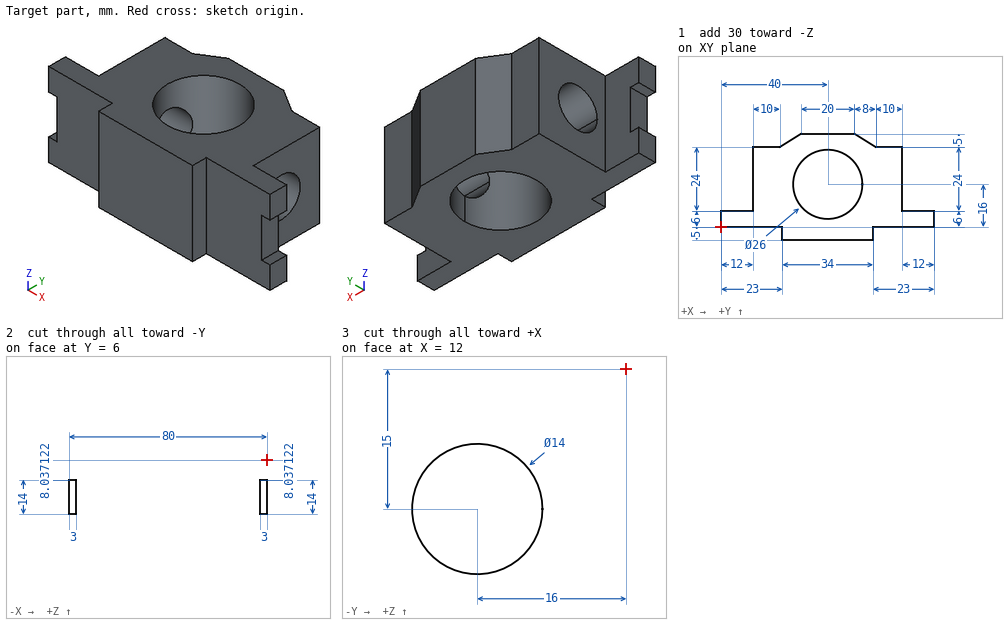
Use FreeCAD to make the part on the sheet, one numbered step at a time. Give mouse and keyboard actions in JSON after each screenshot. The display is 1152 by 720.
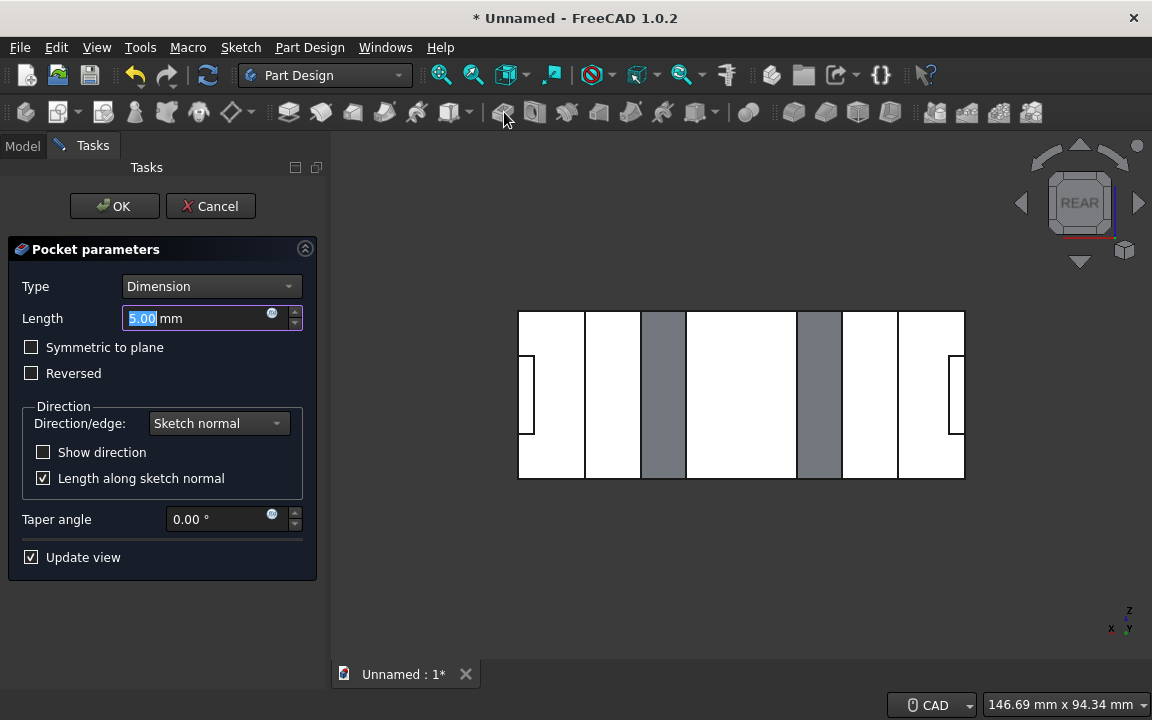
{"action": "left_click", "coordinate": [212, 286]}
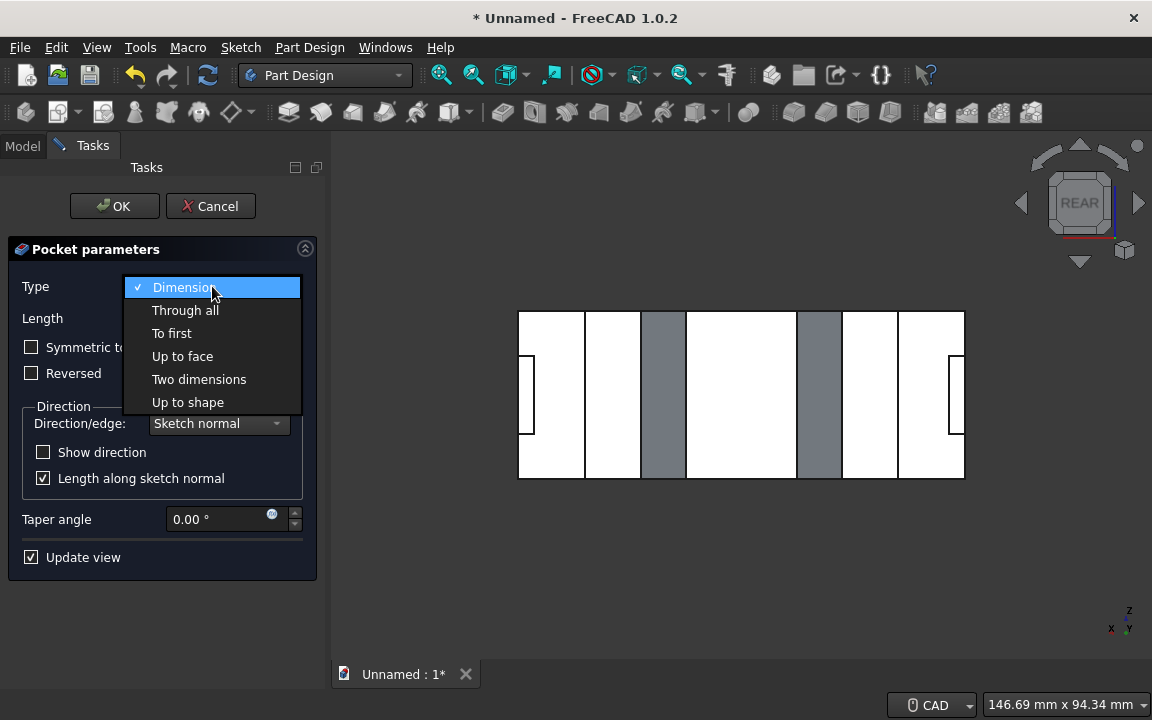
{"action": "left_click", "coordinate": [212, 310]}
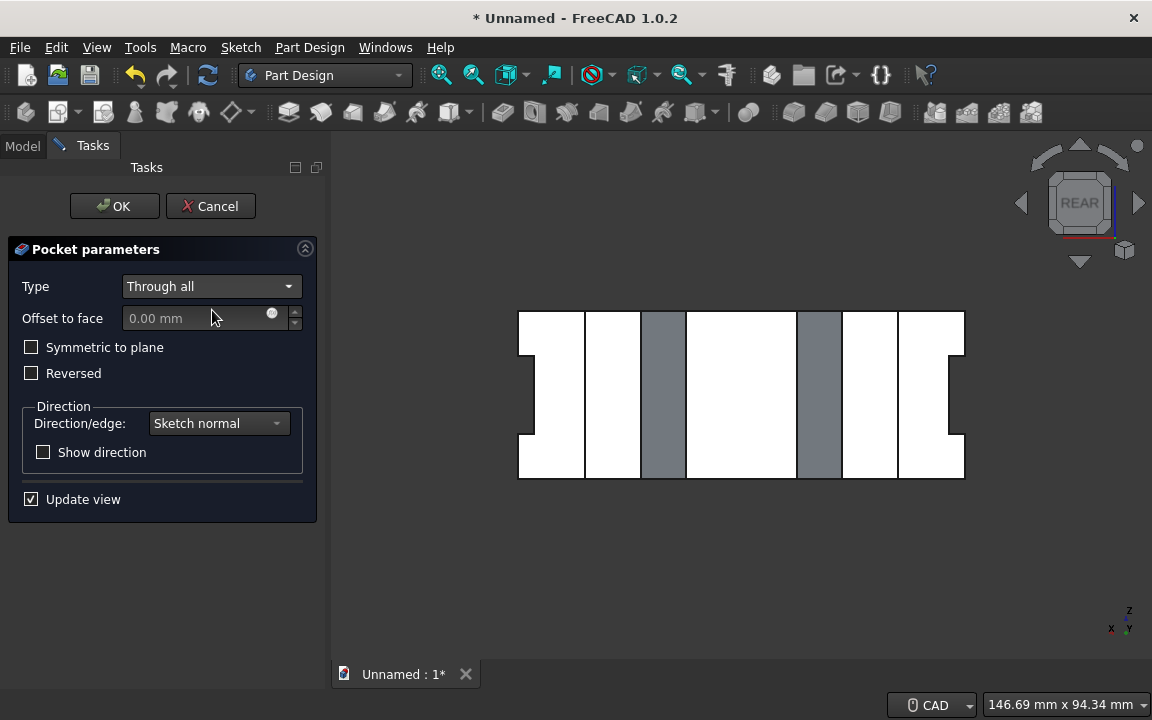
{"action": "left_click", "coordinate": [115, 206]}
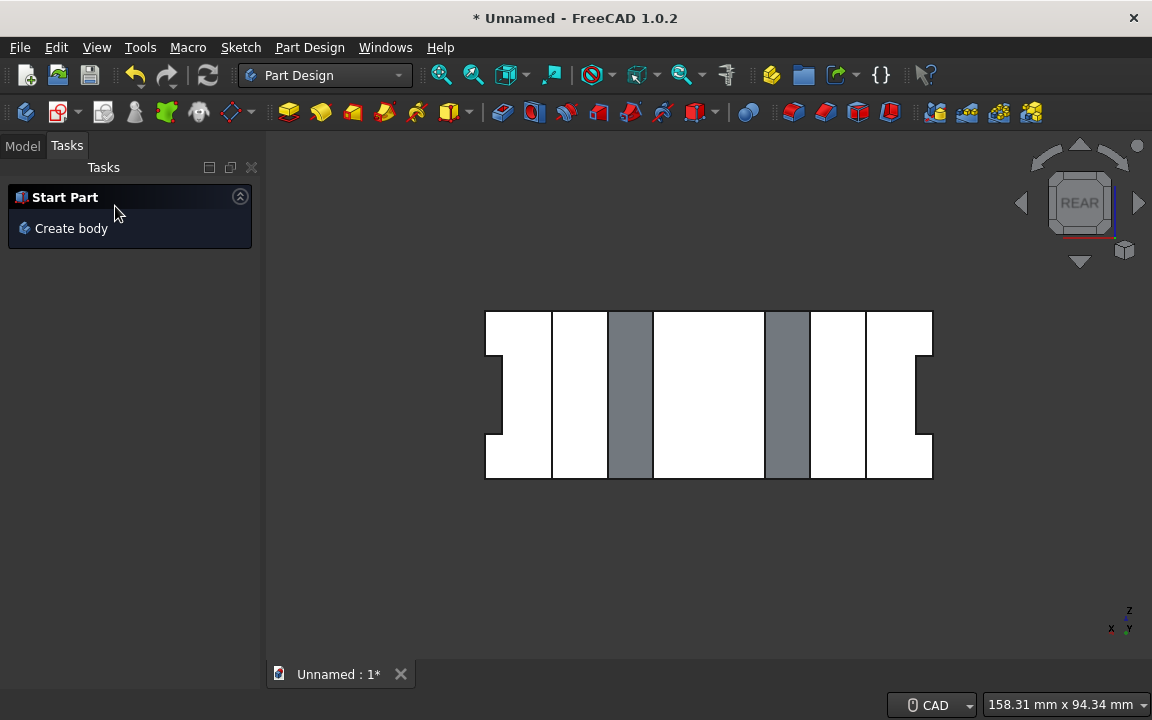
{"action": "key", "text": "6"}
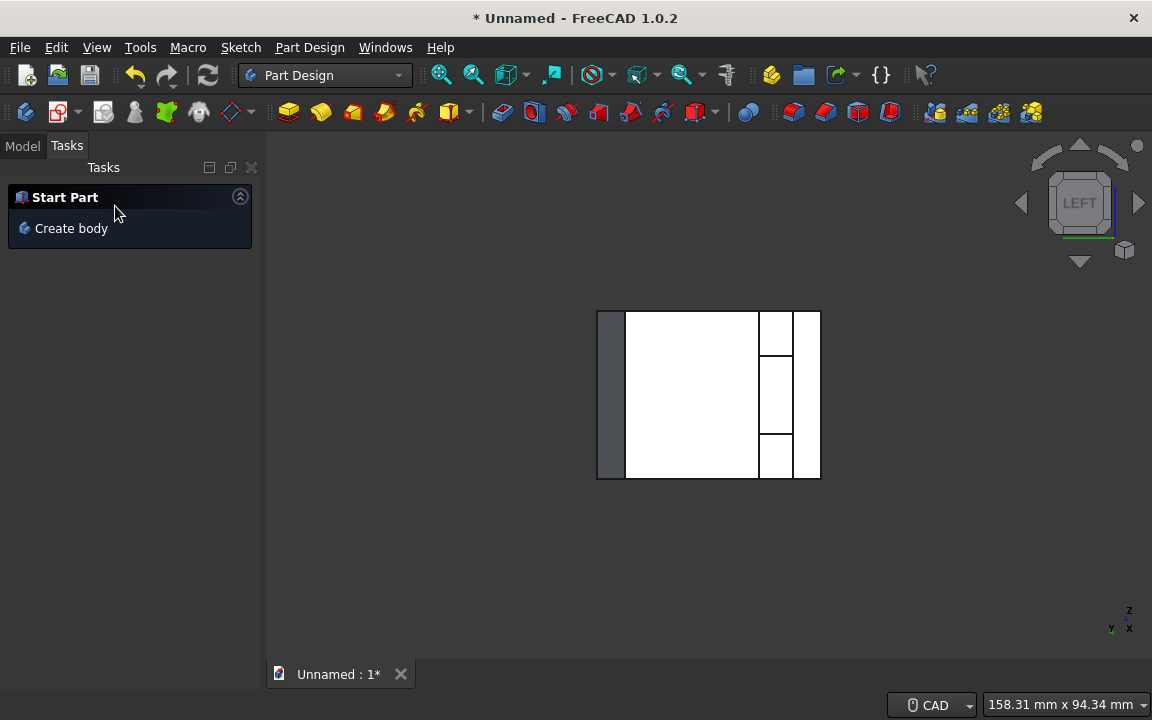
{"action": "left_click", "coordinate": [442, 76]}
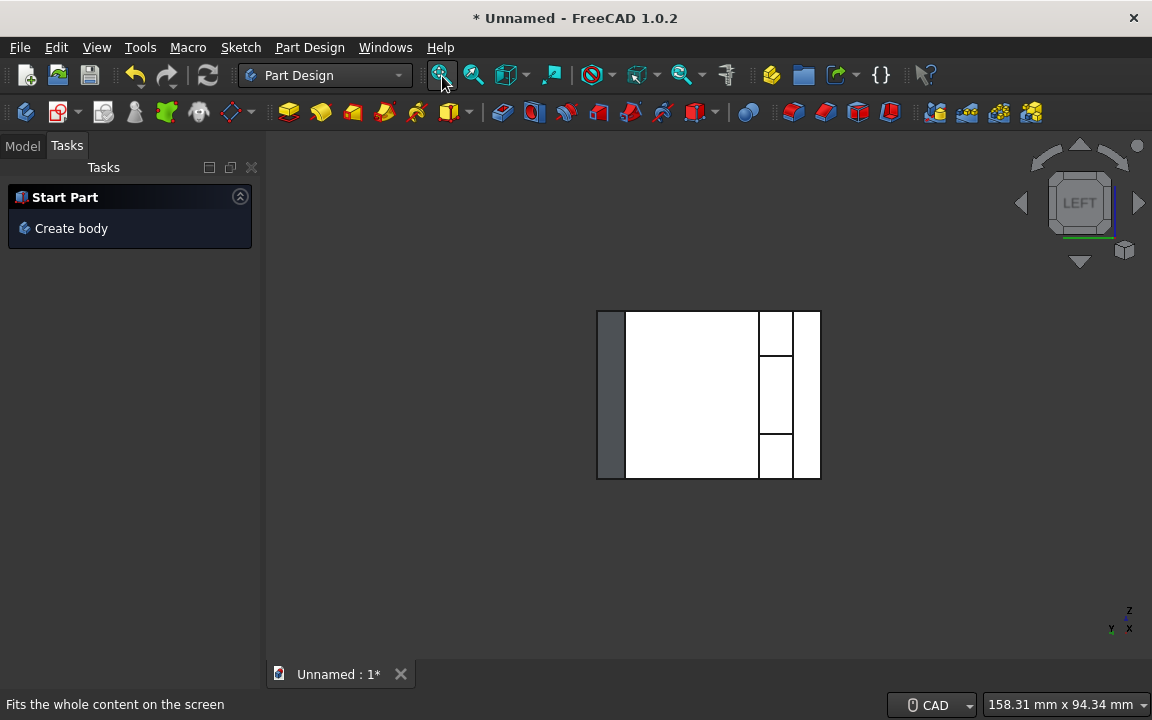
{"action": "left_click", "coordinate": [692, 394]}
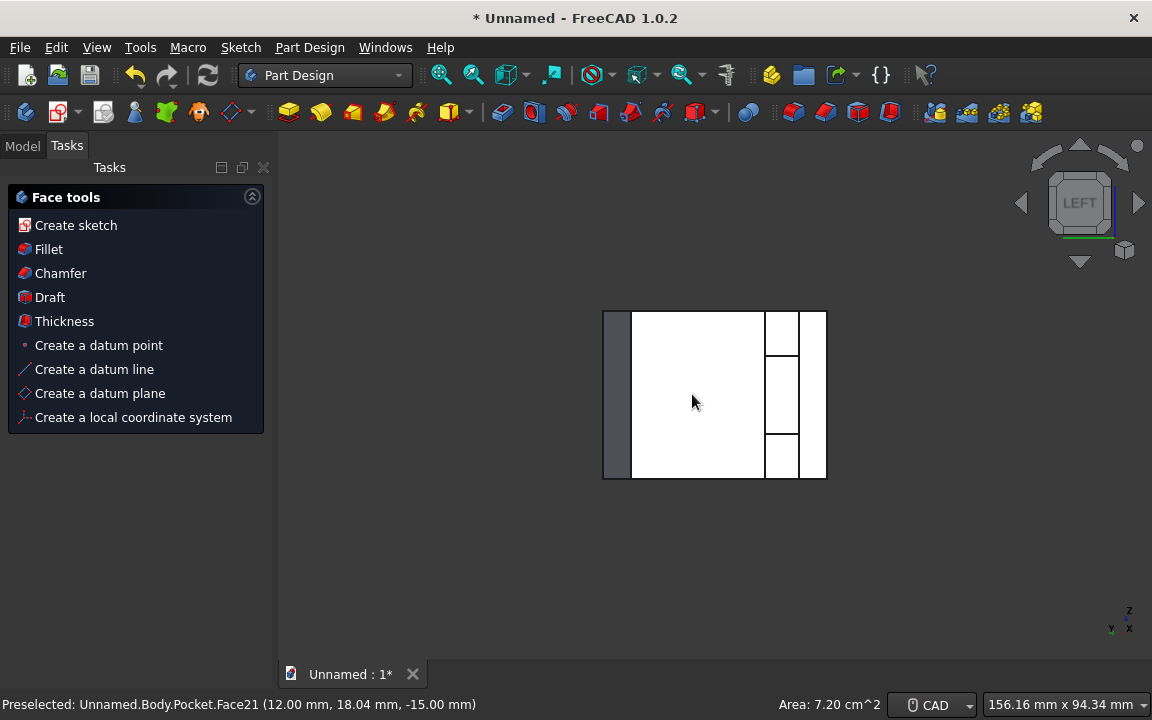
{"action": "left_click", "coordinate": [58, 112]}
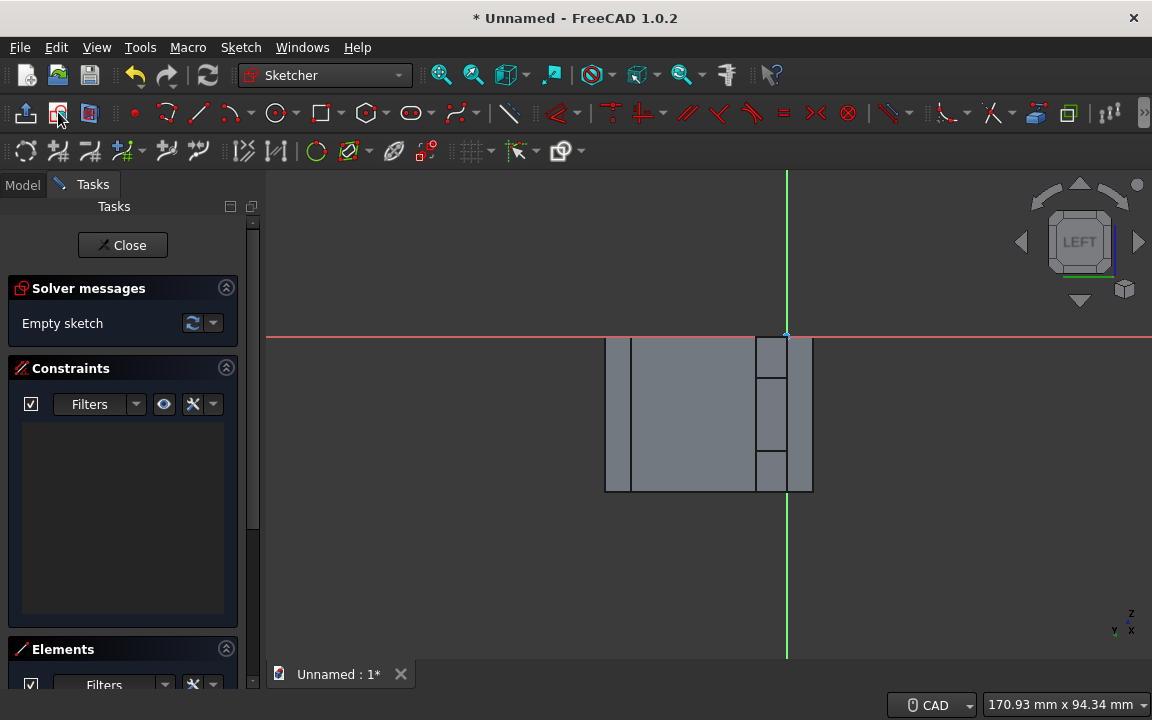
{"action": "left_click", "coordinate": [90, 114]}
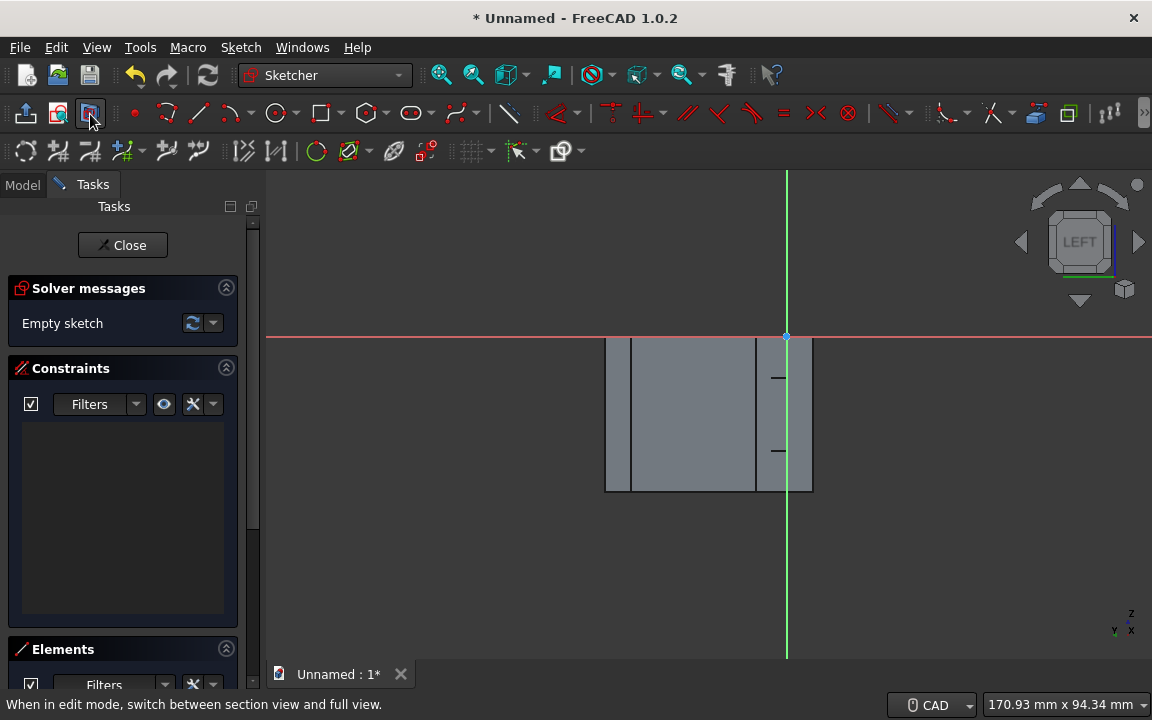
{"action": "scroll", "coordinate": [778, 382], "scroll_direction": "up", "scroll_amount": 5}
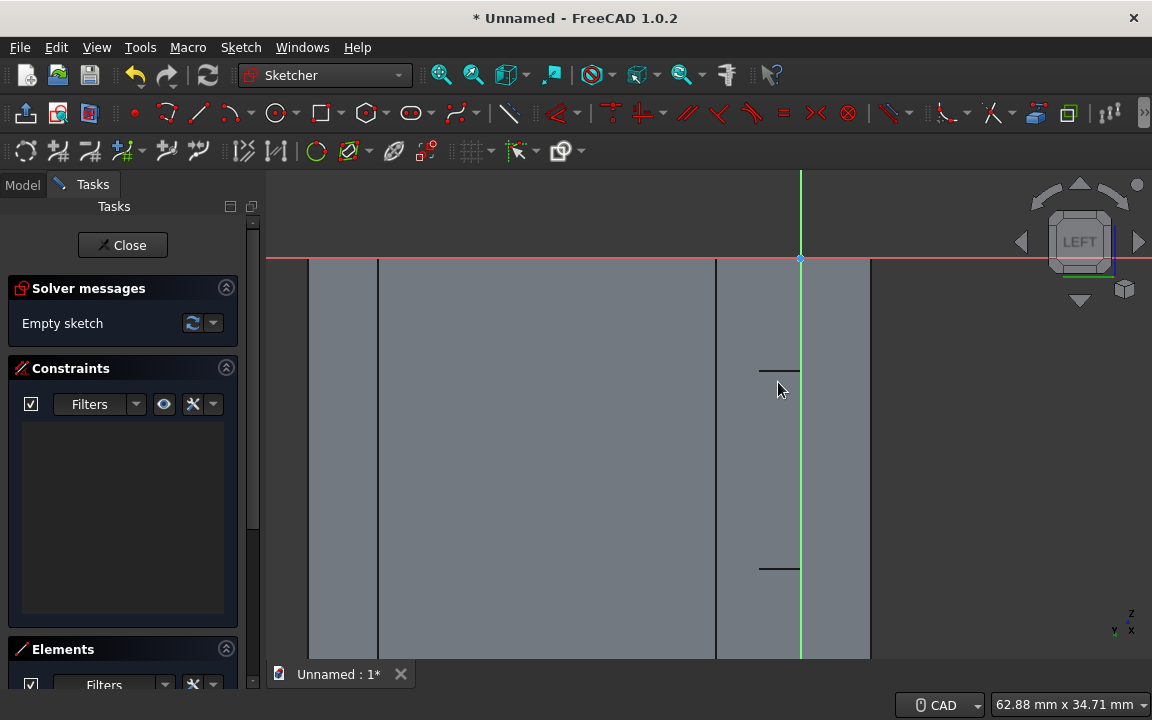
{"action": "left_click", "coordinate": [276, 114]}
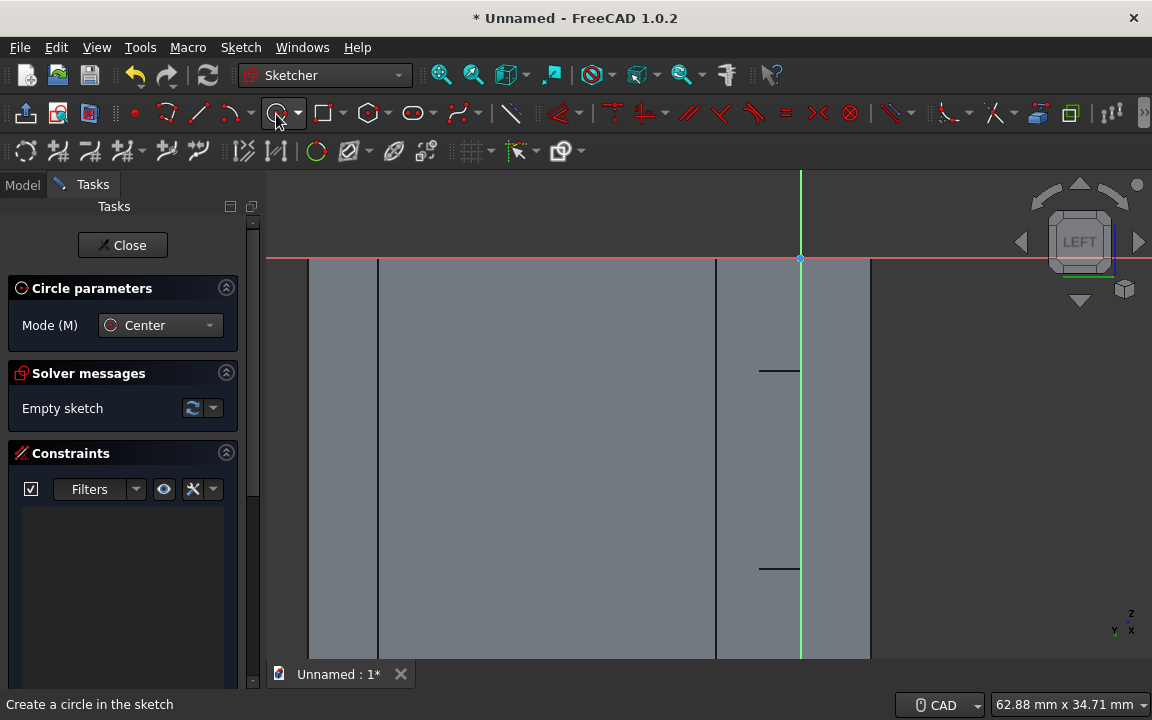
{"action": "left_click", "coordinate": [575, 470]}
{"action": "left_click", "coordinate": [645, 400]}
{"action": "key", "text": "Escape"}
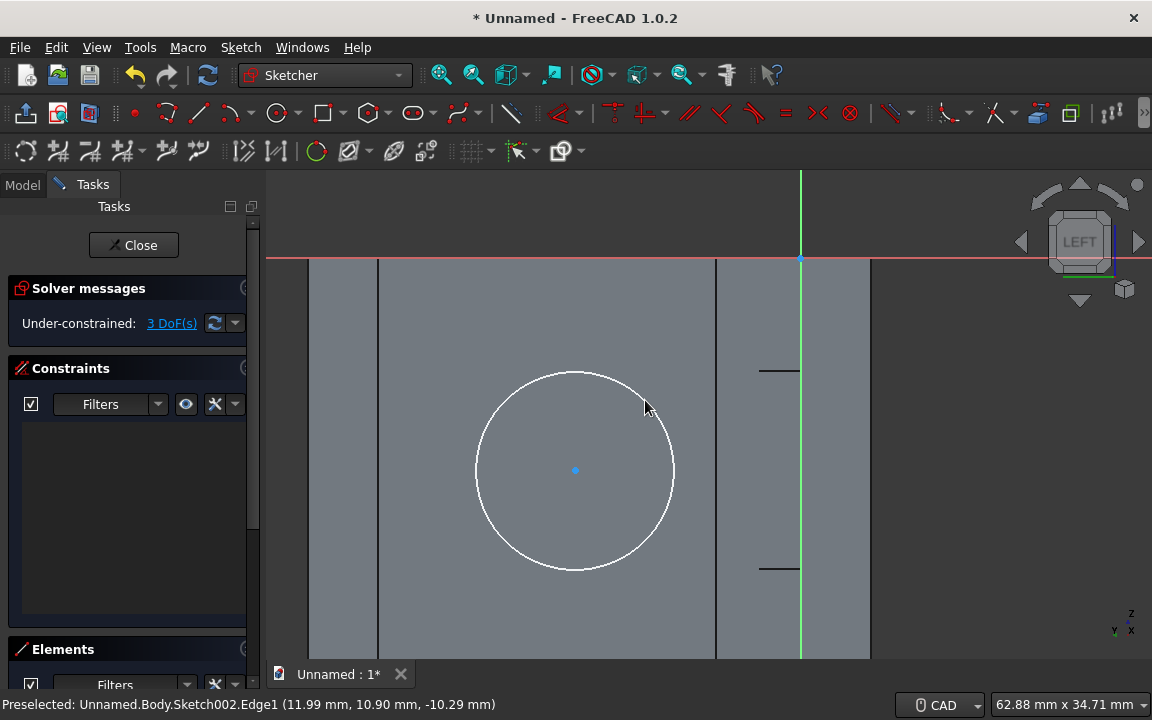
{"action": "key", "text": "d"}